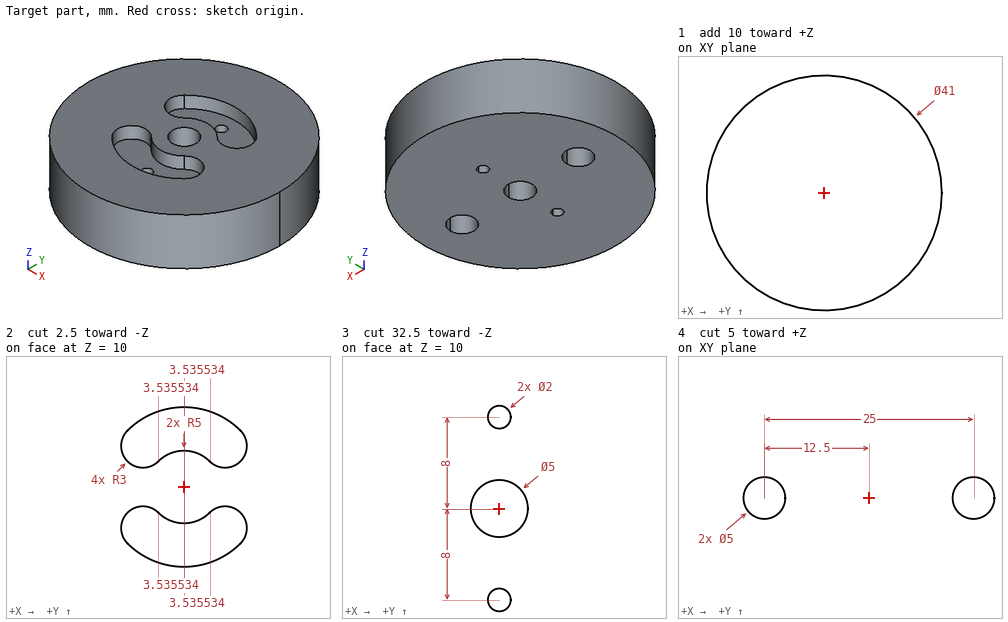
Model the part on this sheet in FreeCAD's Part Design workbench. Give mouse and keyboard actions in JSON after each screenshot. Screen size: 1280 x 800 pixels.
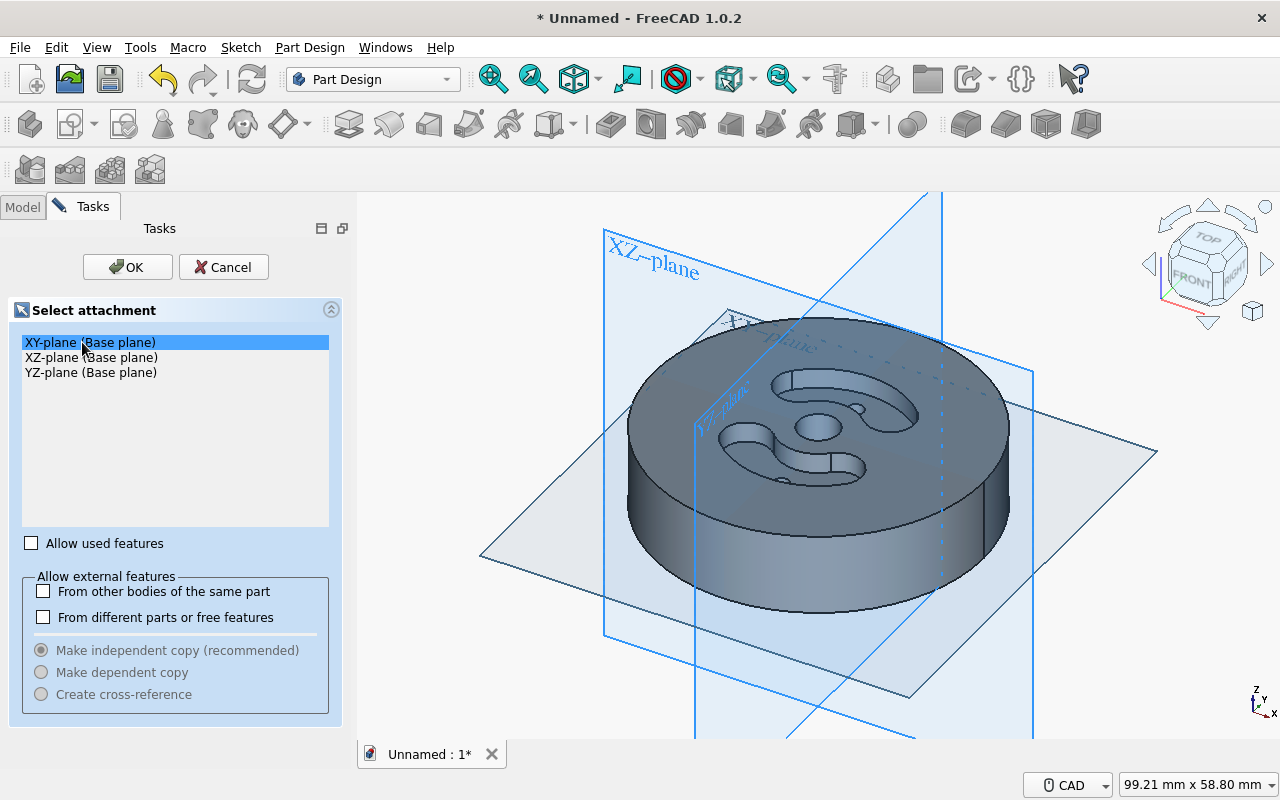
{"action": "left_click", "coordinate": [128, 267]}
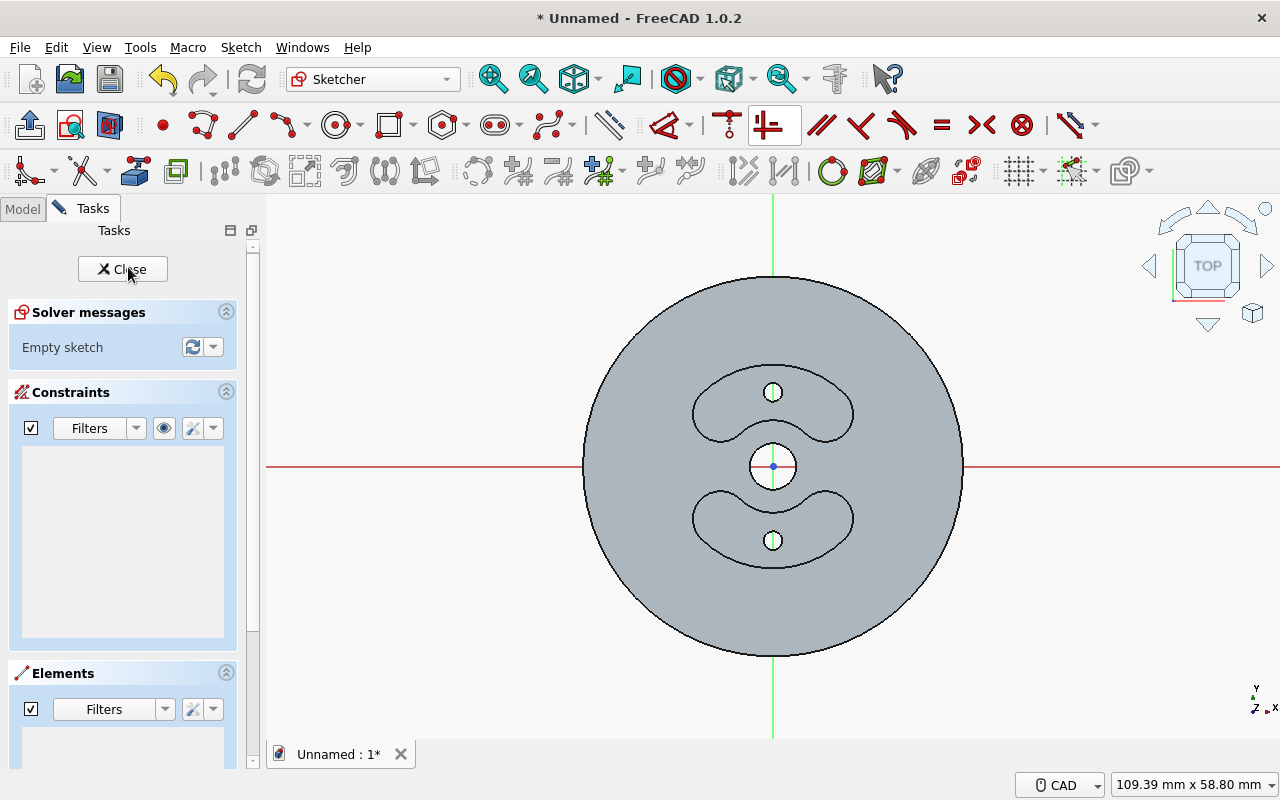
{"action": "key", "text": "q s"}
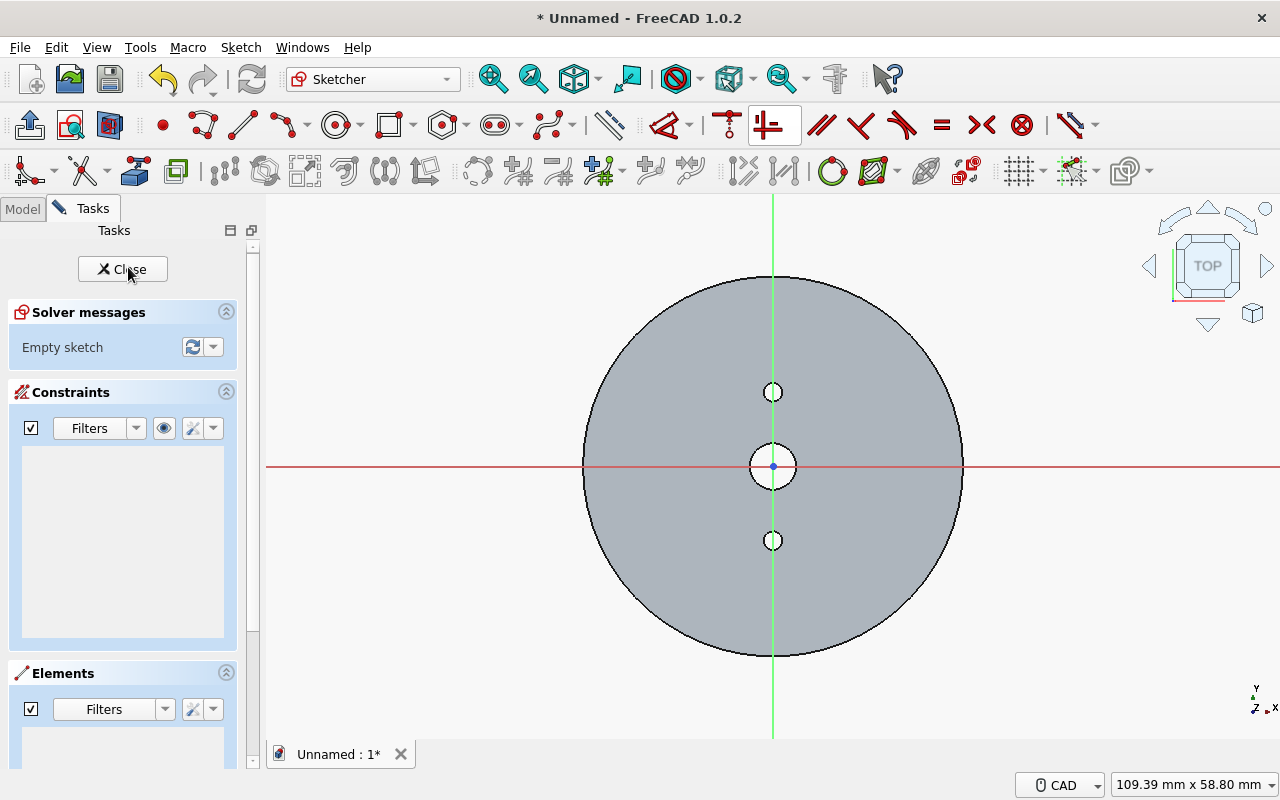
{"action": "scroll", "coordinate": [829, 466], "scroll_direction": "up", "scroll_amount": 4}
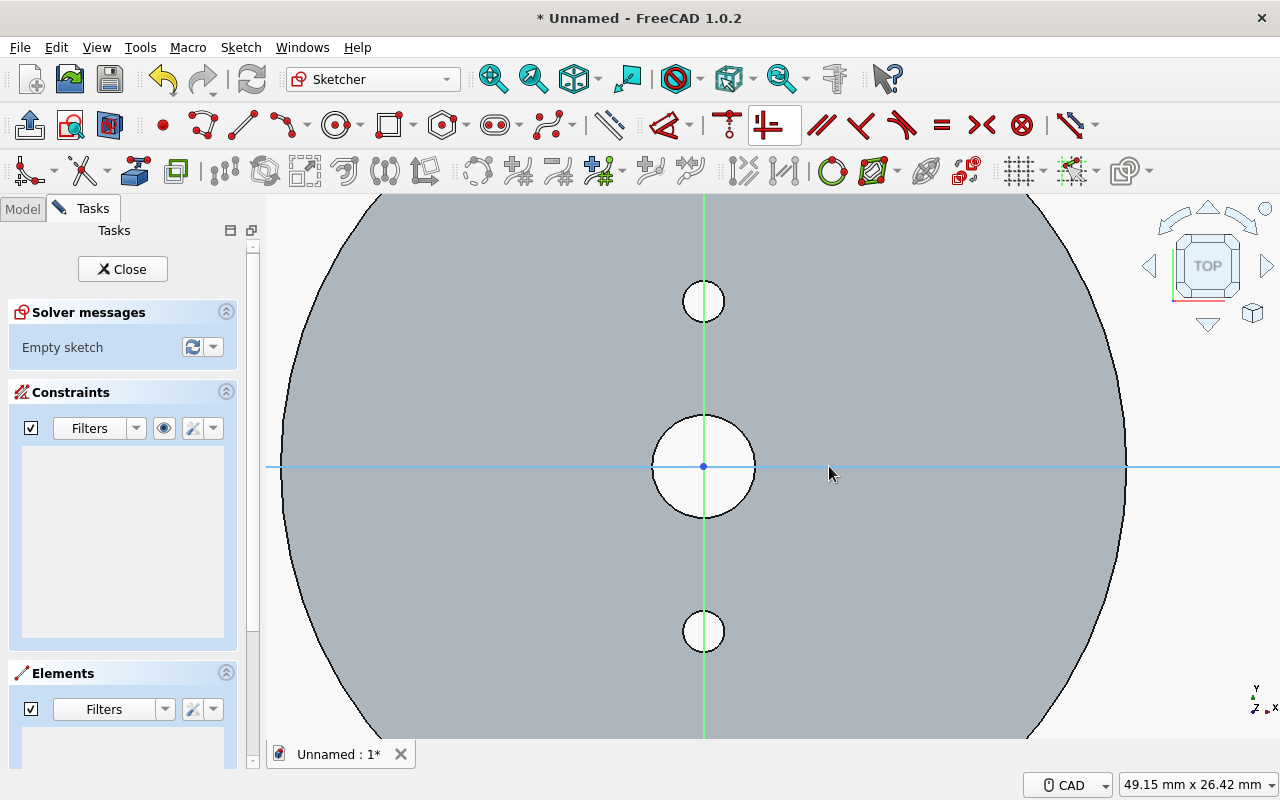
{"action": "key", "text": "g c"}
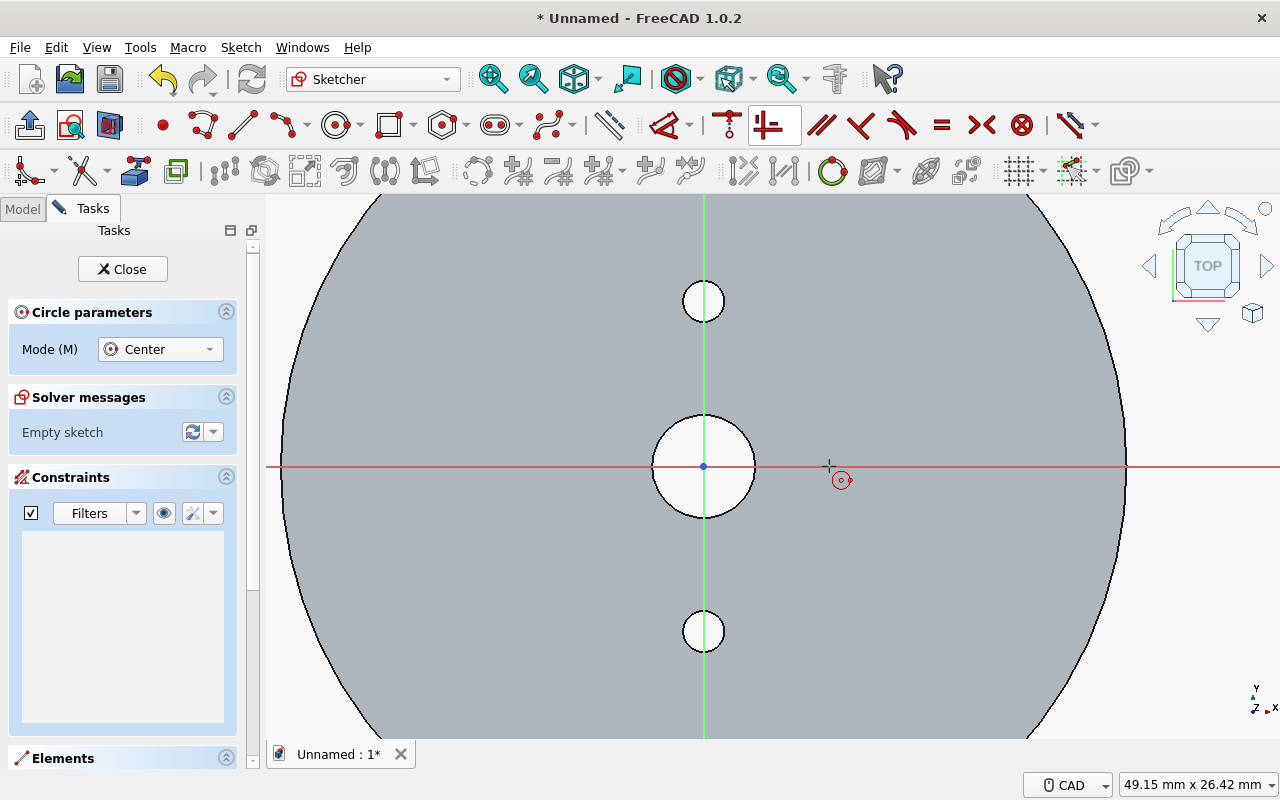
{"action": "left_click", "coordinate": [446, 466]}
{"action": "left_click", "coordinate": [482, 430]}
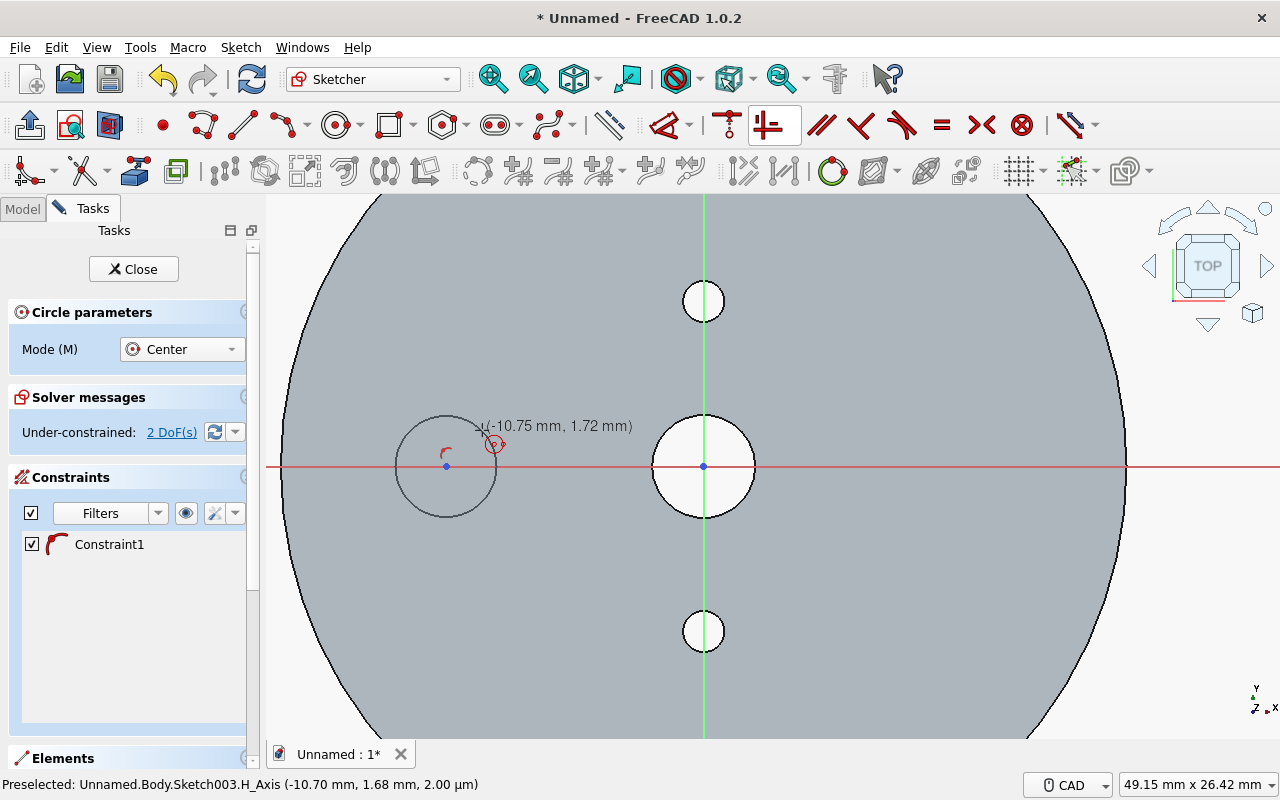
{"action": "left_click", "coordinate": [962, 466]}
{"action": "left_click", "coordinate": [998, 430]}
{"action": "key", "text": "Escape"}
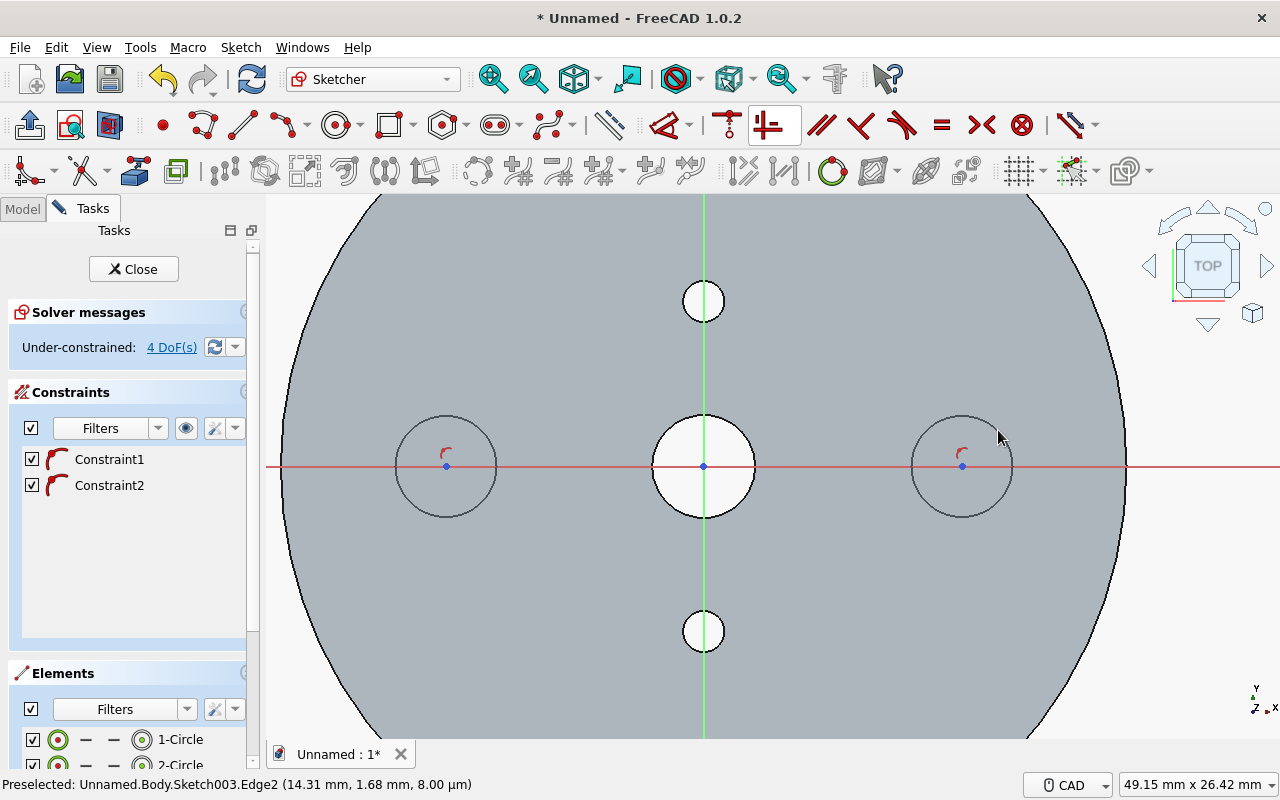
{"action": "left_click", "coordinate": [482, 431]}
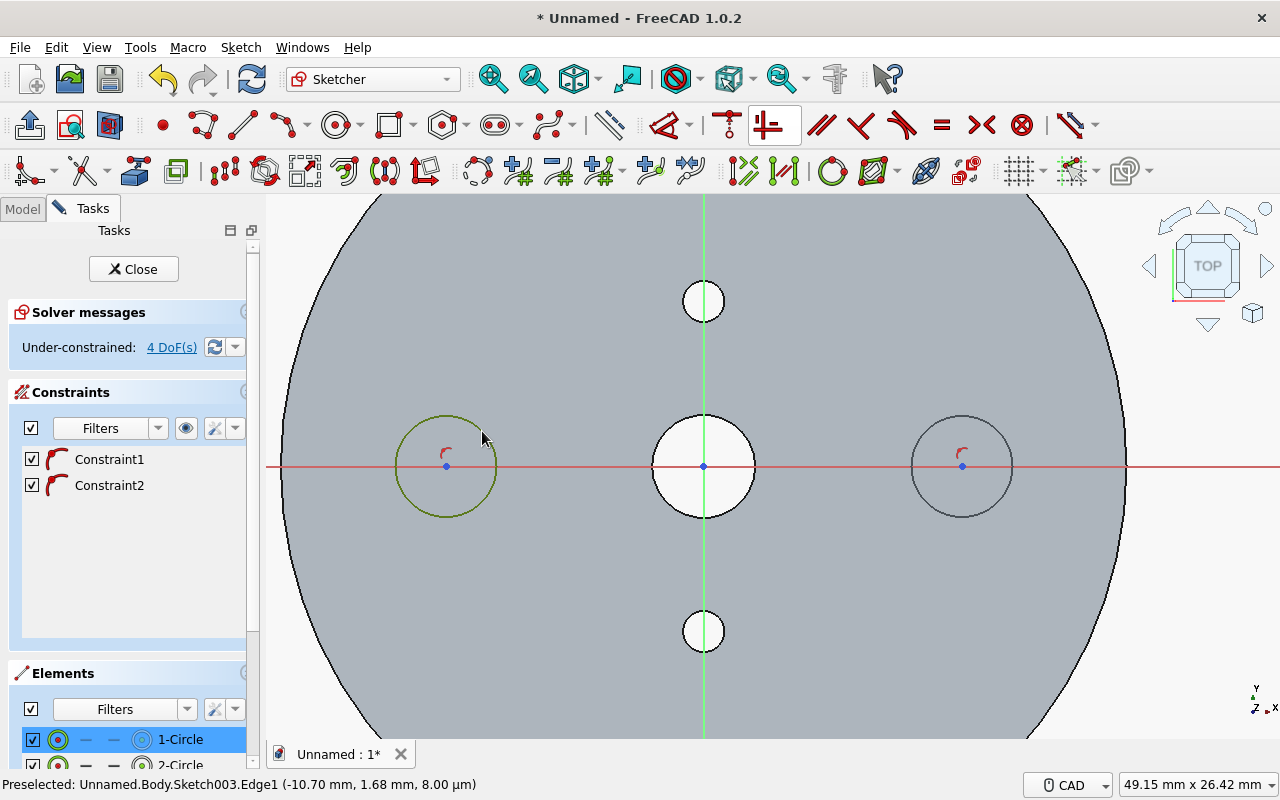
{"action": "left_click", "coordinate": [998, 431]}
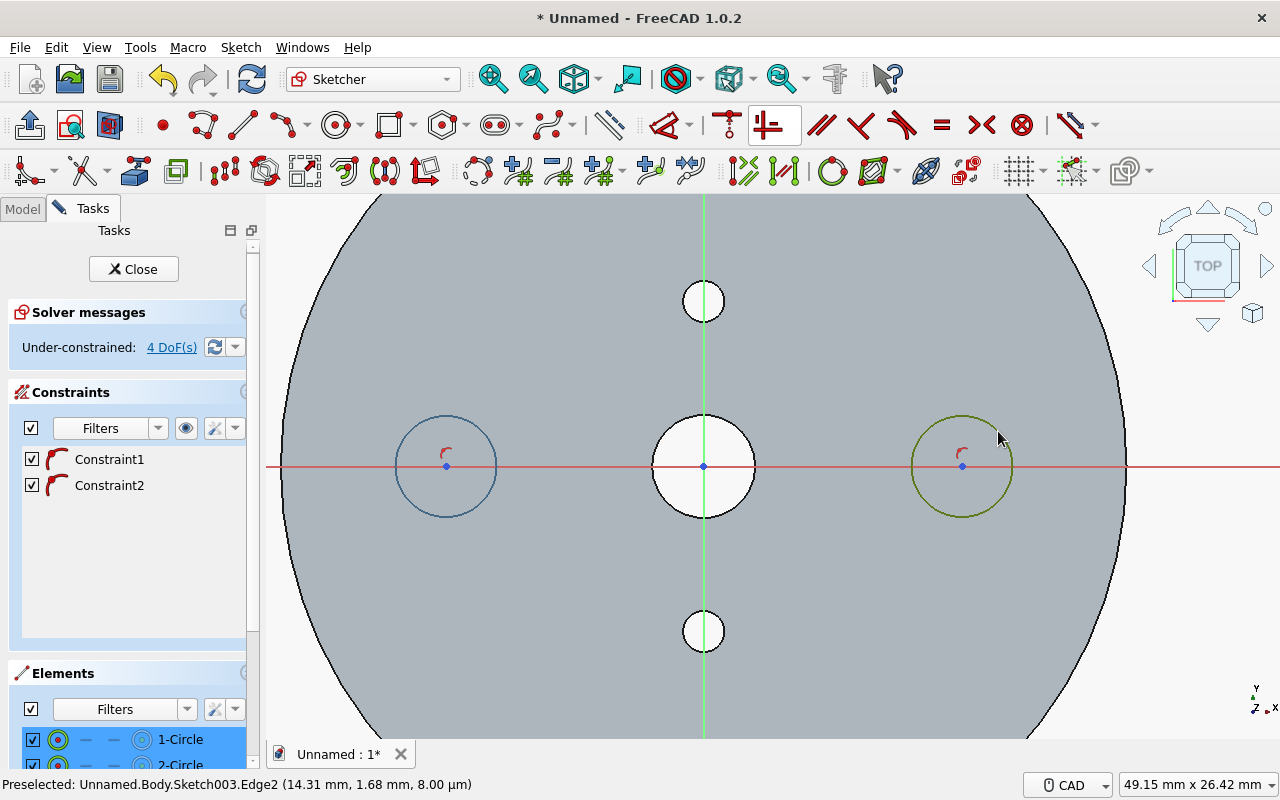
{"action": "key", "text": "e"}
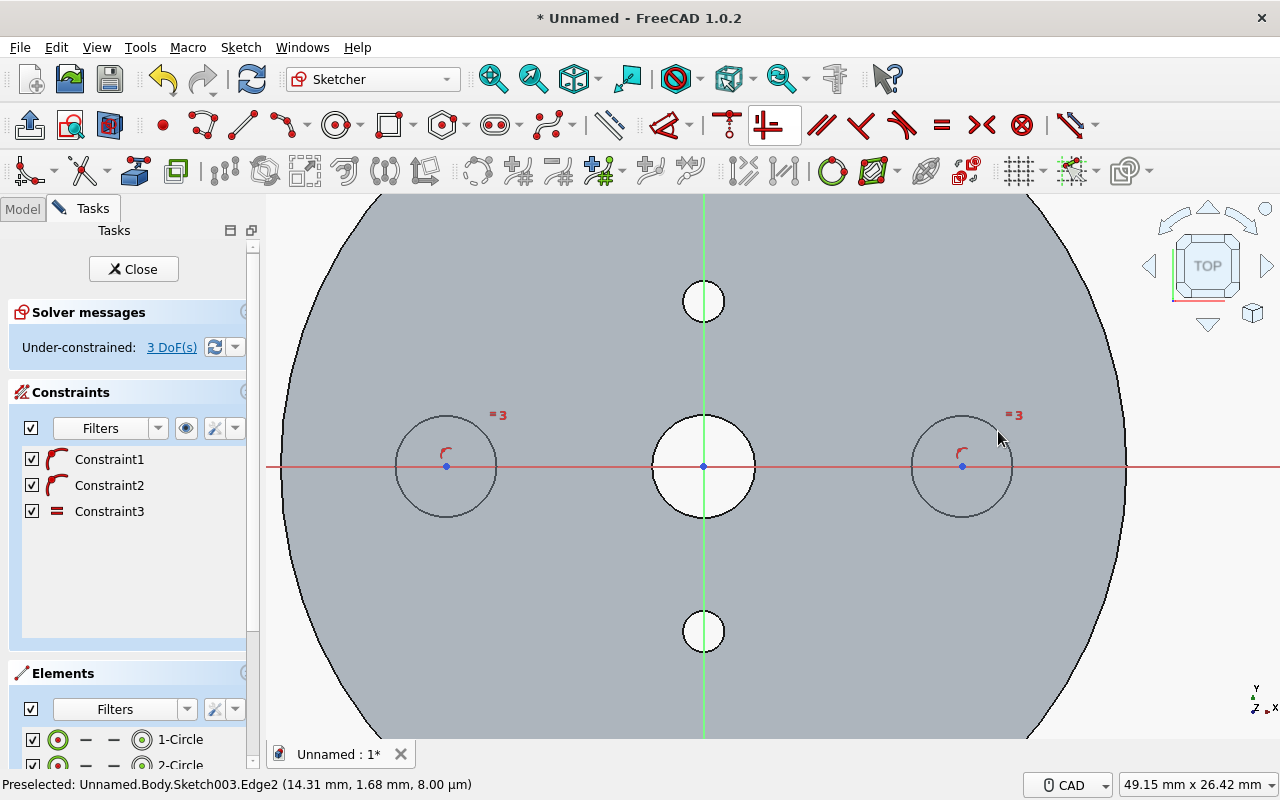
{"action": "key", "text": "d"}